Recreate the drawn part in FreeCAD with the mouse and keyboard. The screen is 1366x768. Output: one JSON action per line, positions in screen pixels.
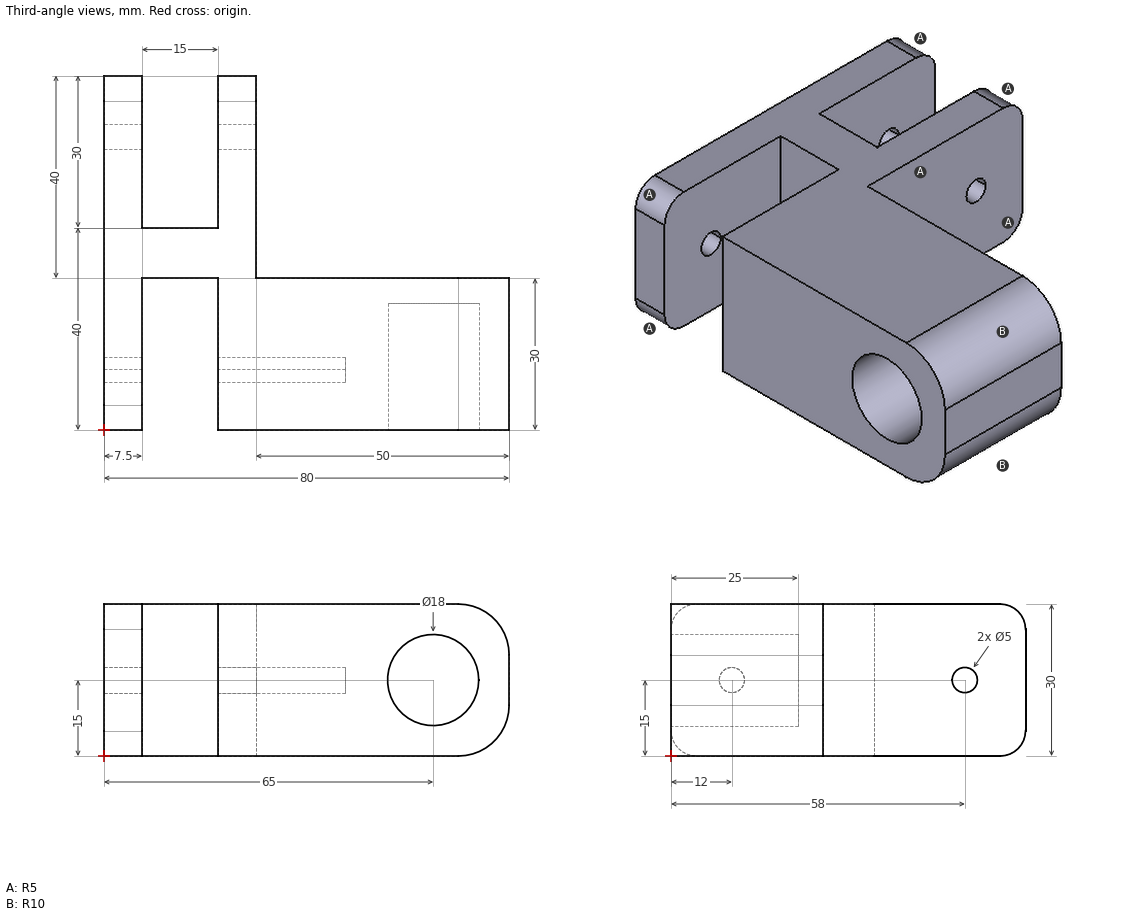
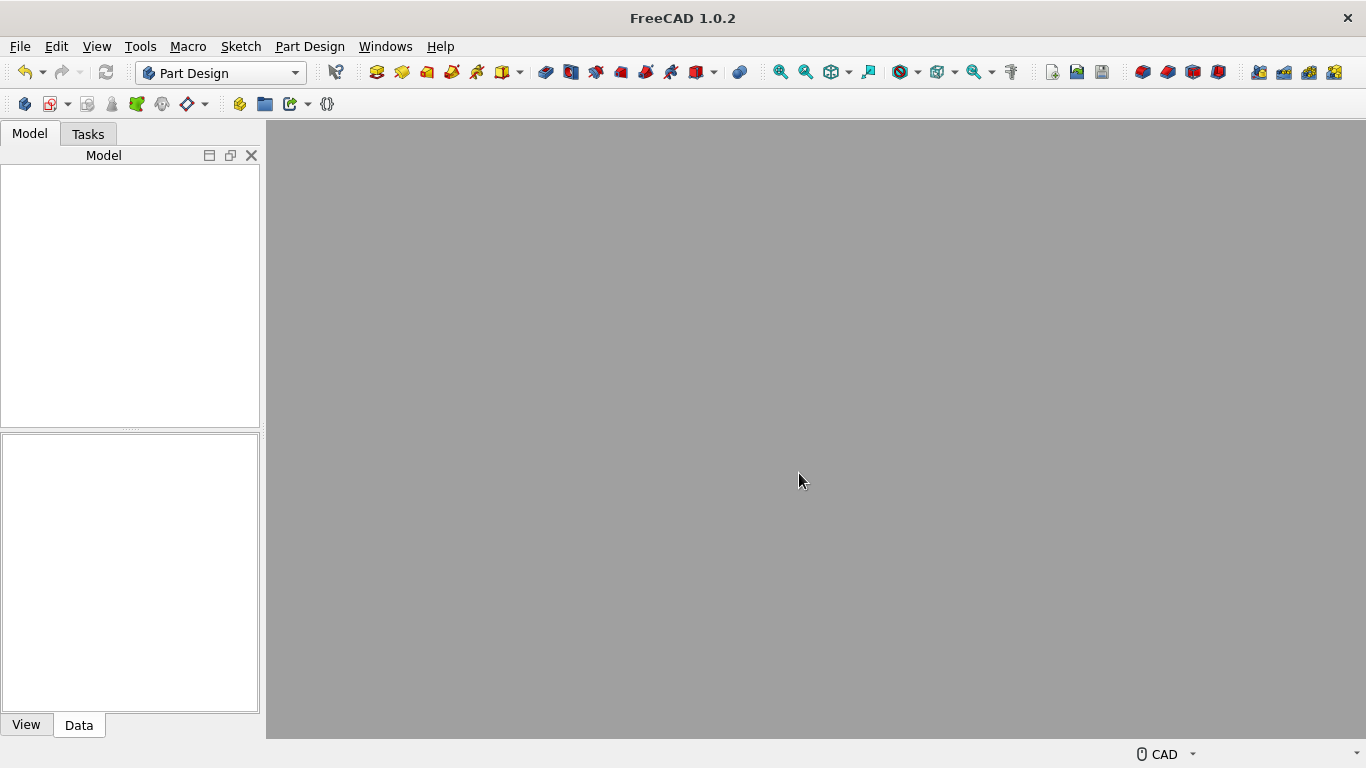
{"action": "key", "text": "ctrl+n"}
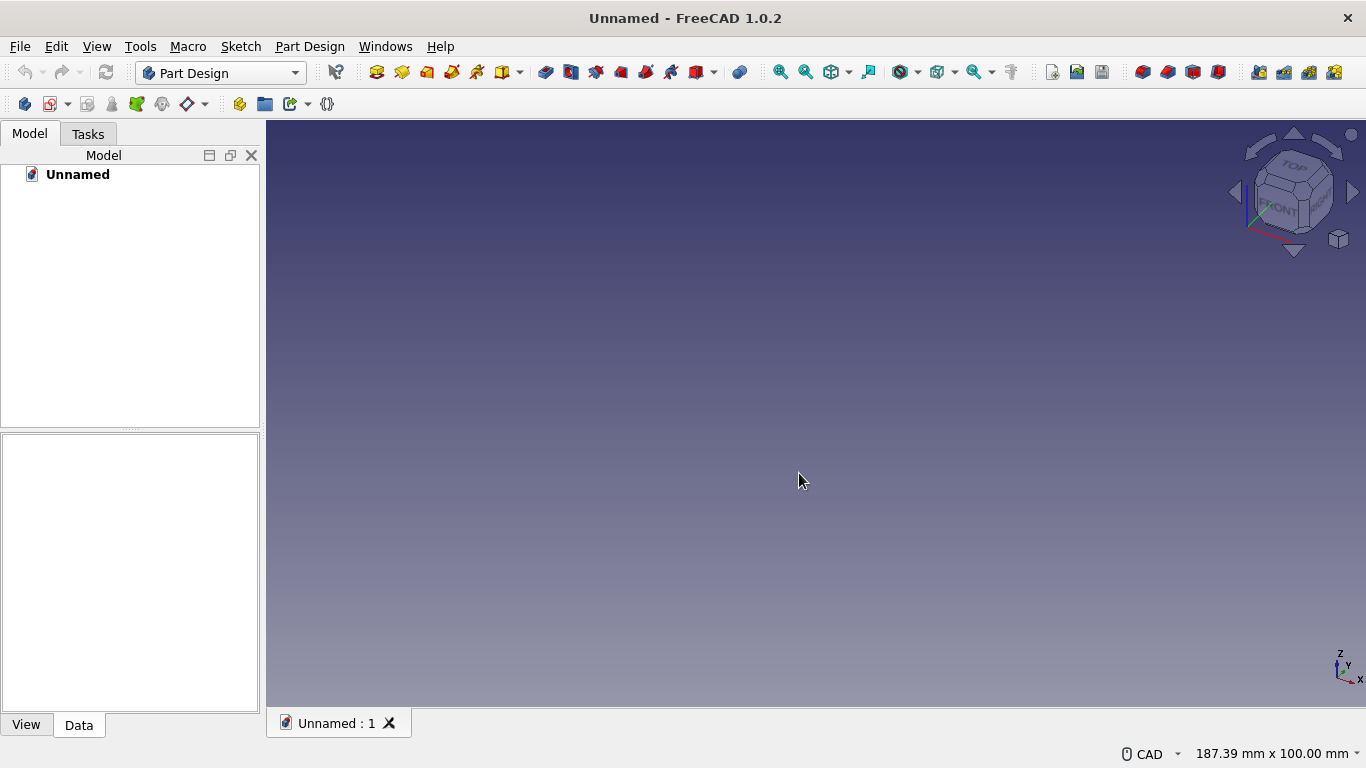
{"action": "left_click", "coordinate": [50, 104]}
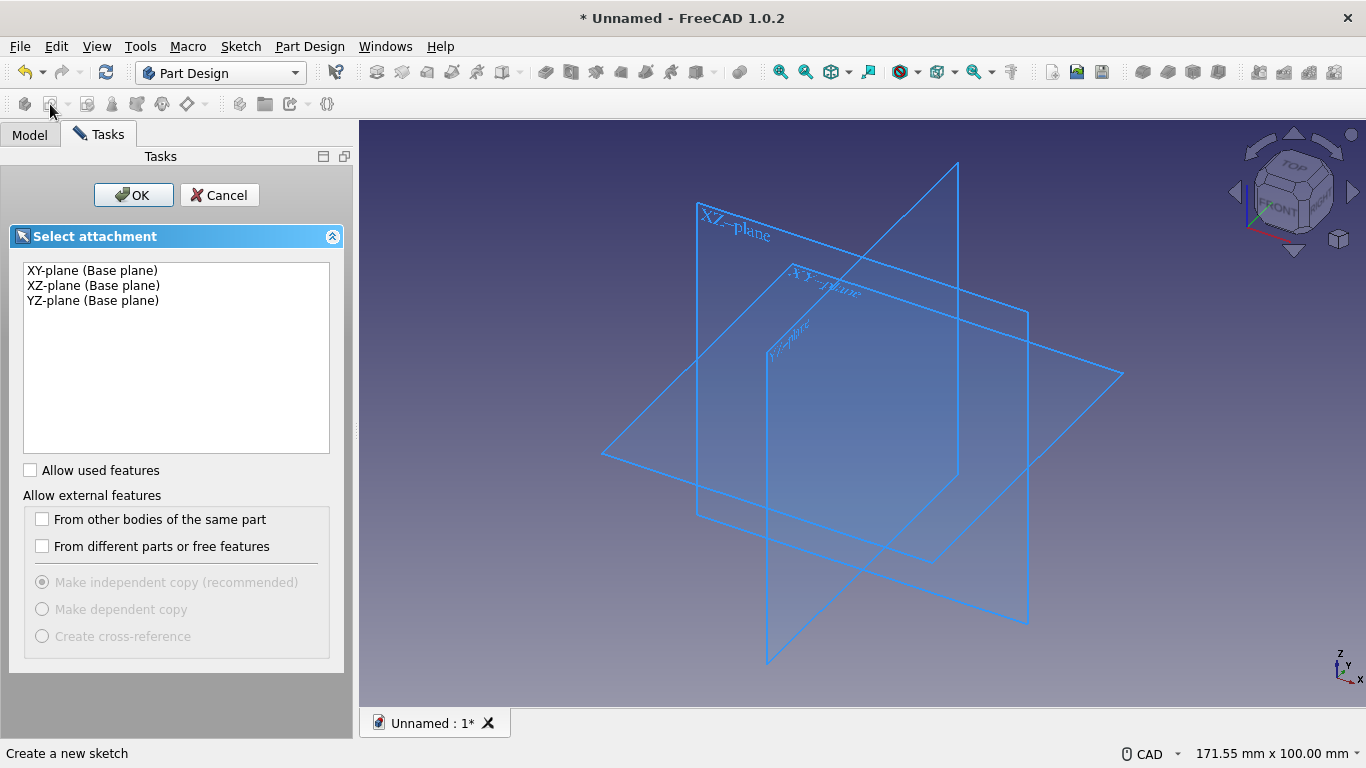
{"action": "left_click", "coordinate": [84, 270]}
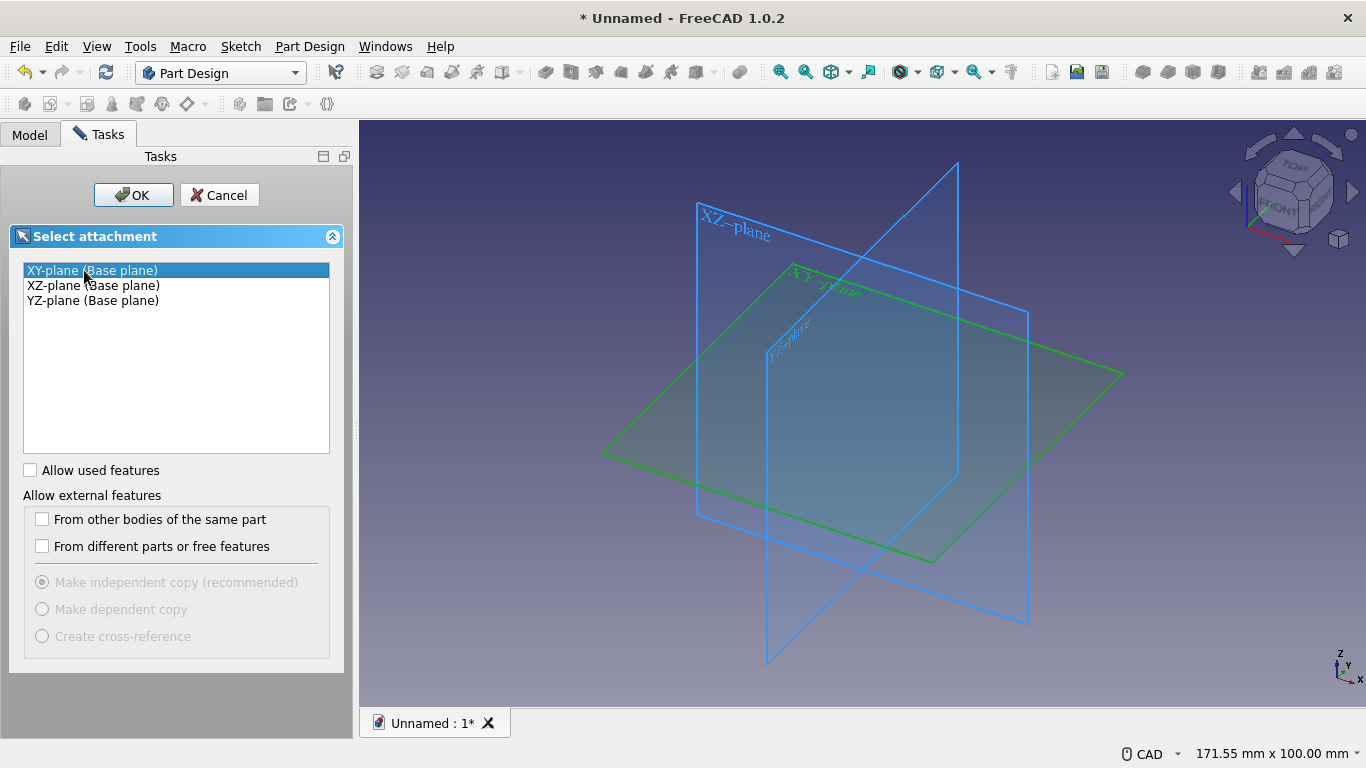
{"action": "left_click", "coordinate": [134, 195]}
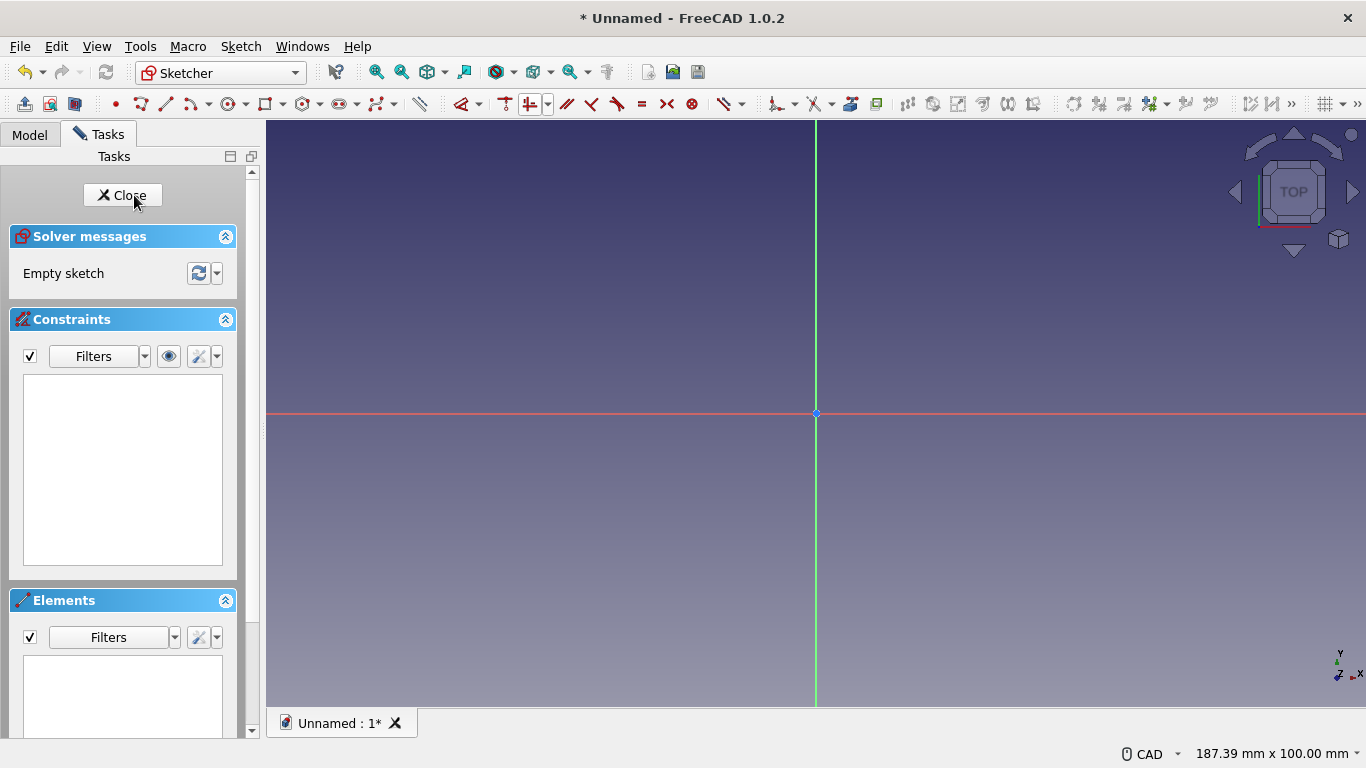
{"action": "scroll", "coordinate": [294, 679], "scroll_direction": "down", "scroll_amount": 2}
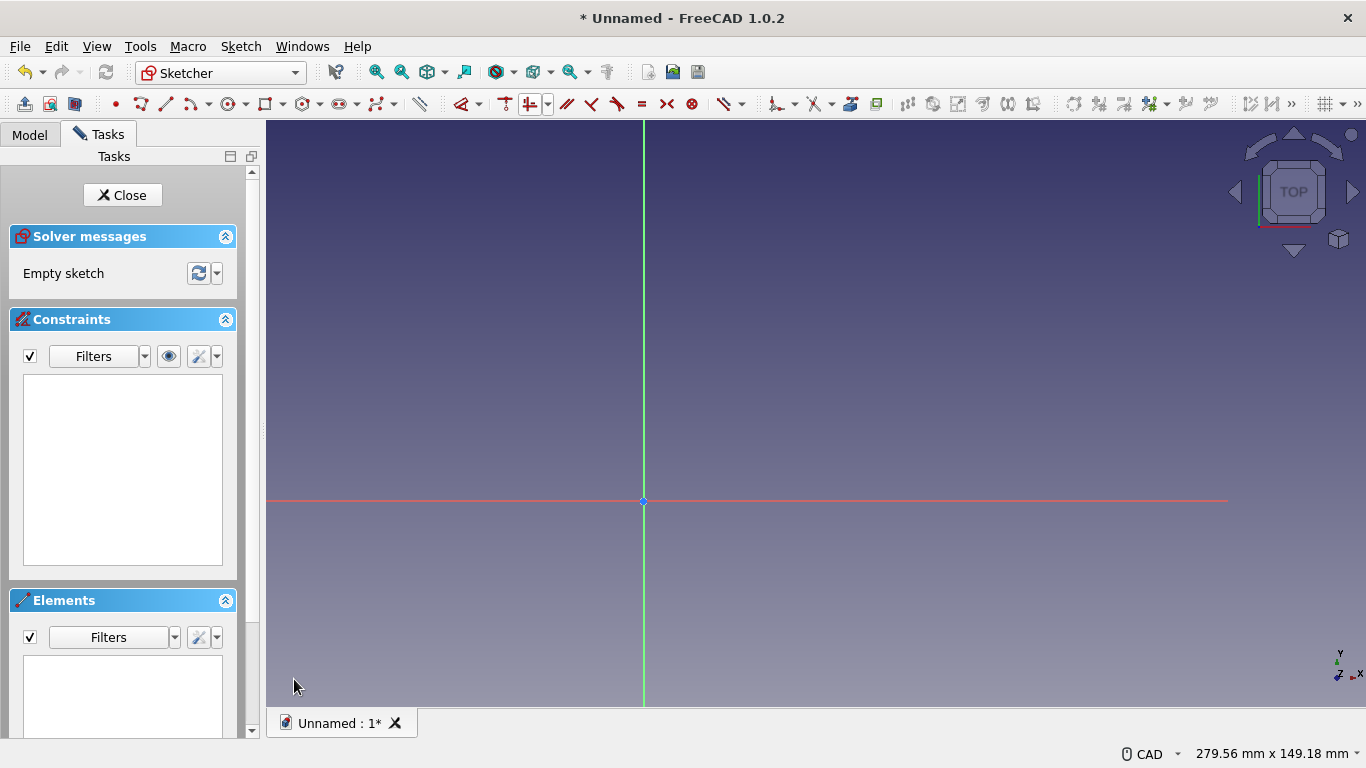
{"action": "scroll", "coordinate": [911, 262], "scroll_direction": "up", "scroll_amount": 2}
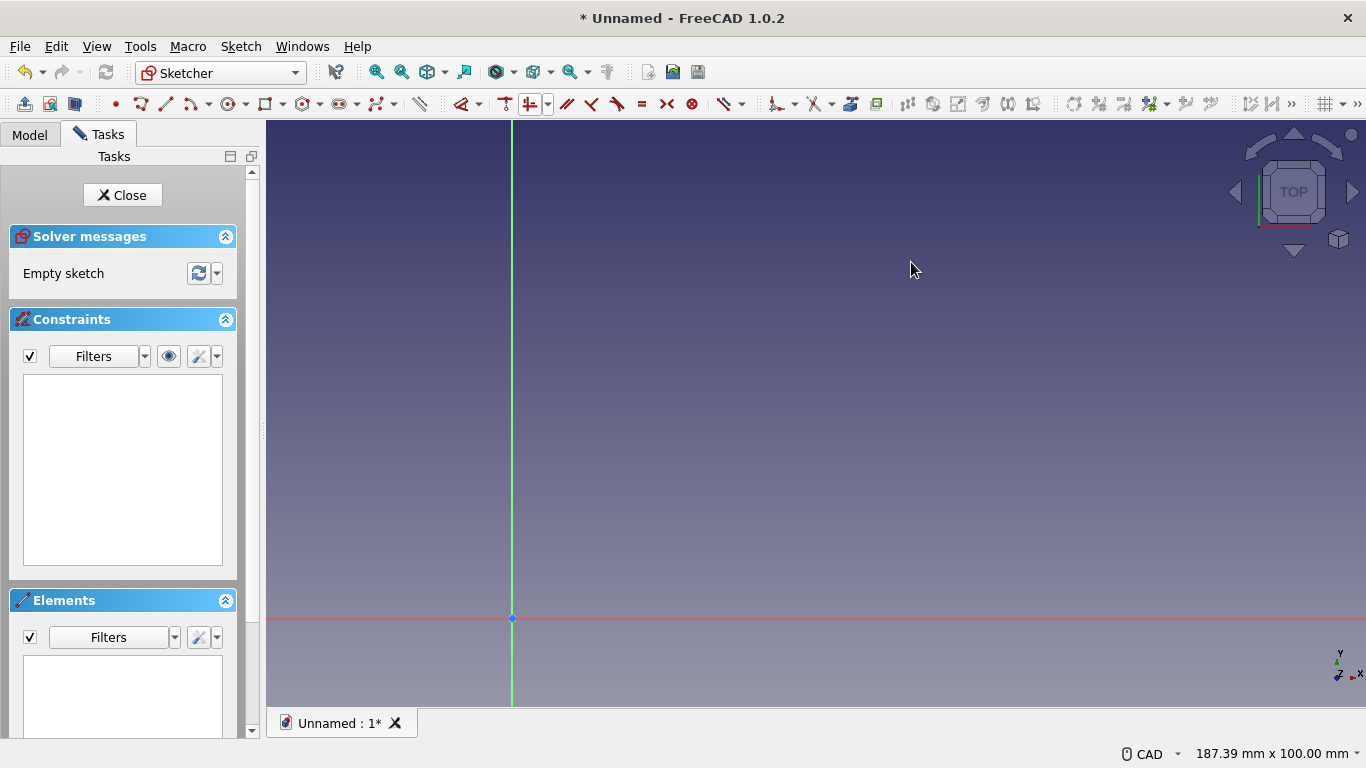
{"action": "left_click", "coordinate": [141, 104]}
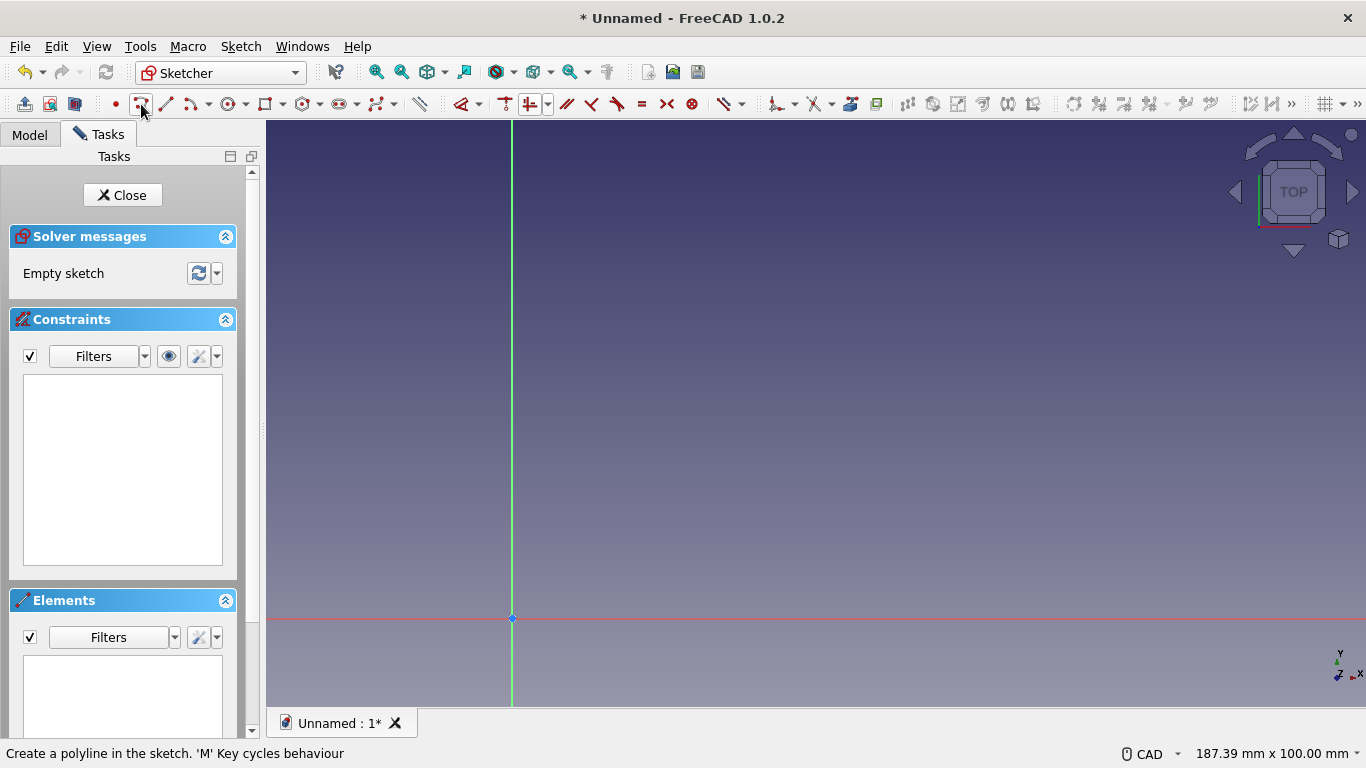
{"action": "left_click", "coordinate": [512, 619]}
{"action": "left_click", "coordinate": [982, 610]}
{"action": "left_click", "coordinate": [982, 443]}
{"action": "left_click", "coordinate": [688, 443]}
{"action": "left_click", "coordinate": [688, 208]}
{"action": "left_click", "coordinate": [521, 208]}
{"action": "left_click", "coordinate": [512, 619]}
{"action": "key", "text": "Escape"}
{"action": "key", "text": "Escape"}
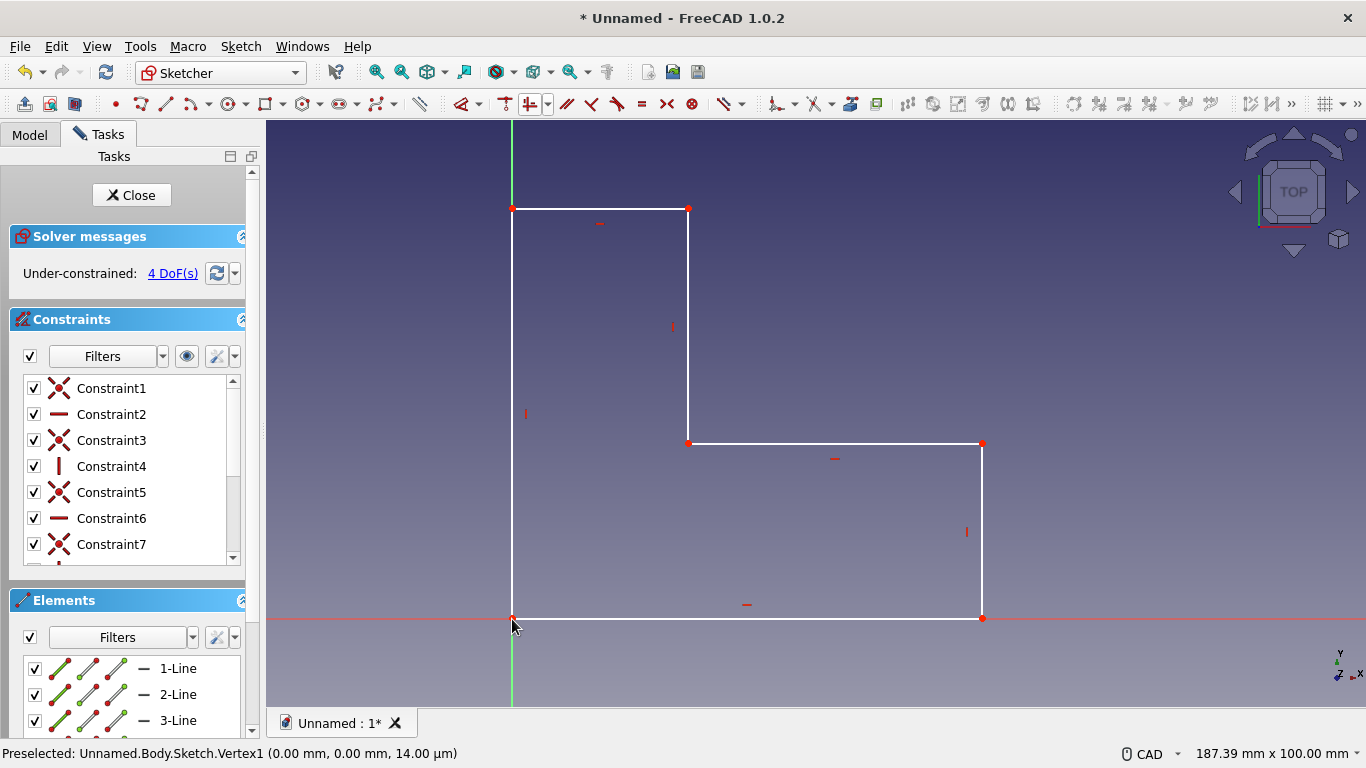
{"action": "key", "text": "d"}